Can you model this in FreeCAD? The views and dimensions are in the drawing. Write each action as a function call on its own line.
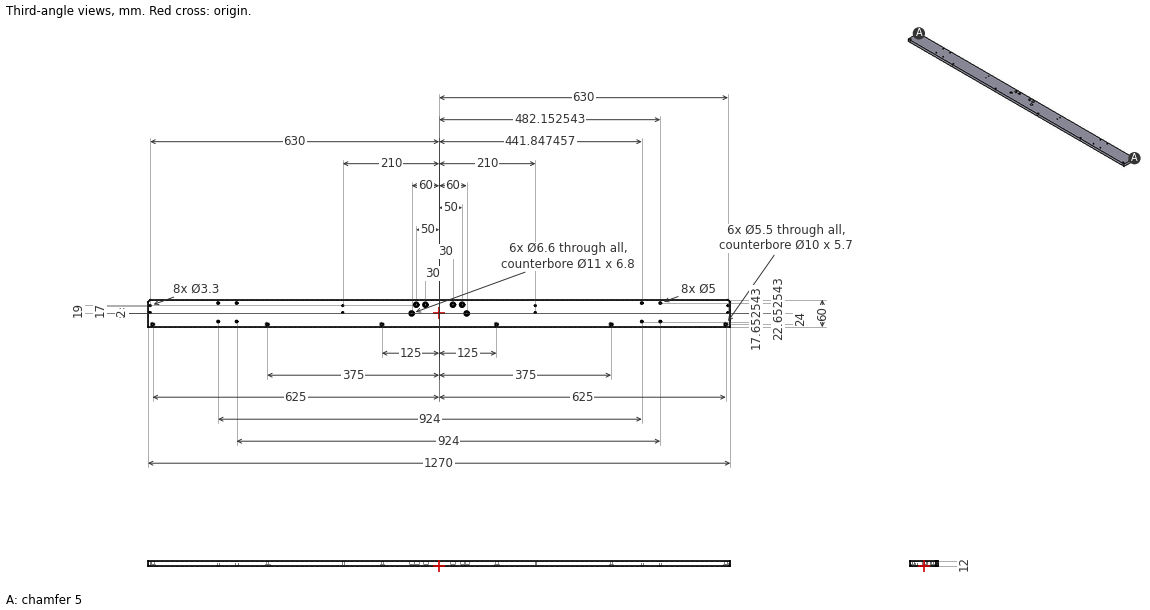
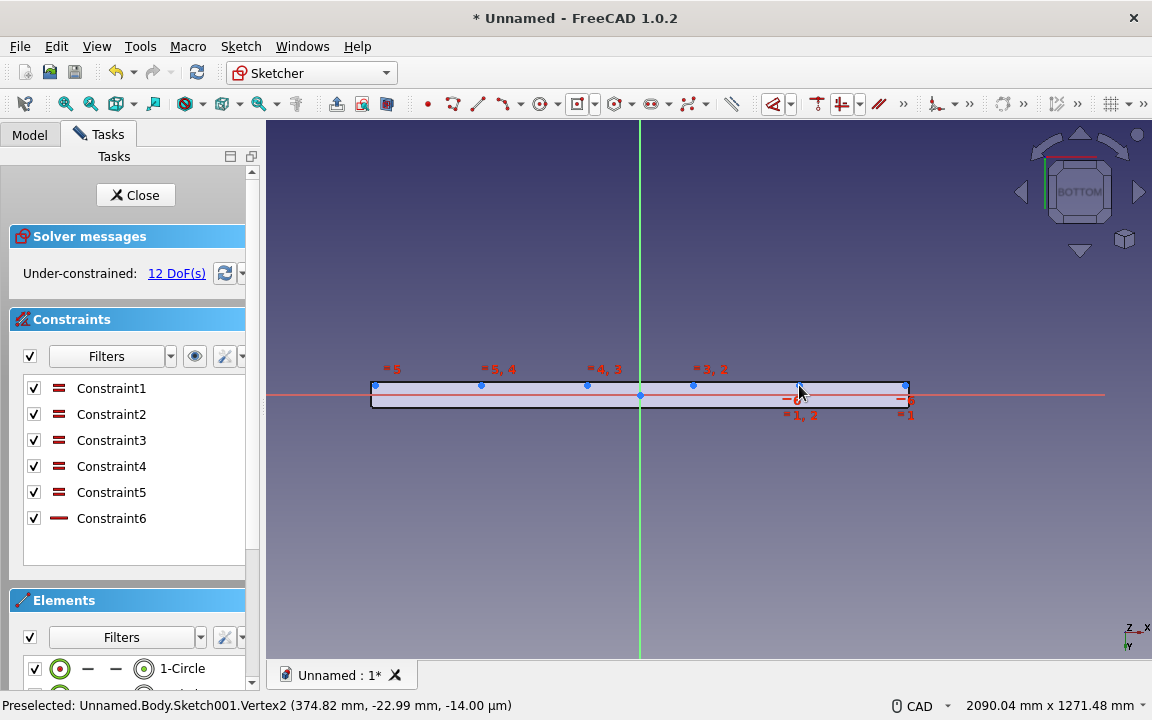
click(799, 386)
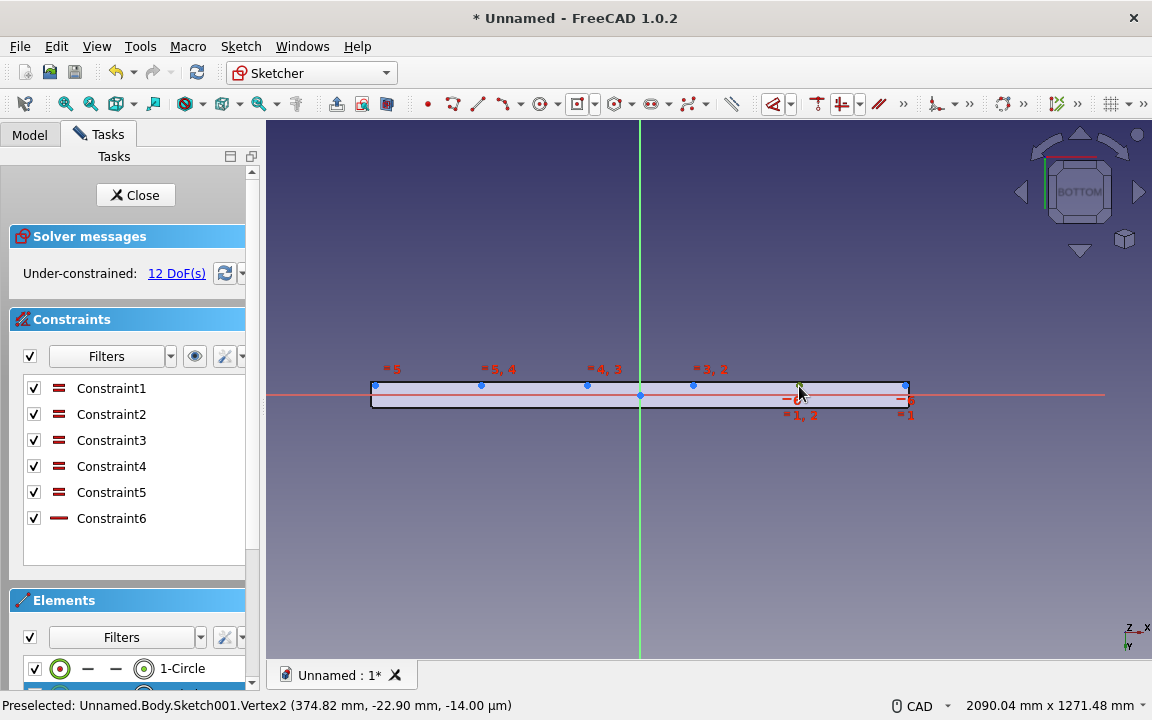
click(693, 385)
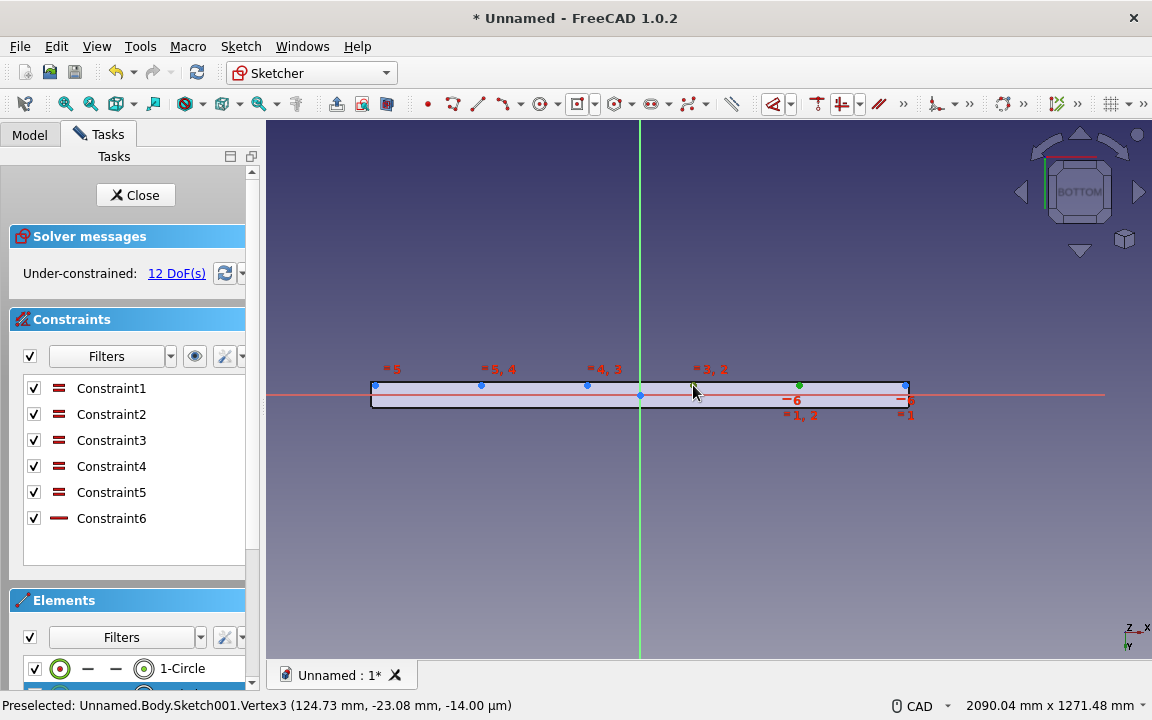
click(860, 104)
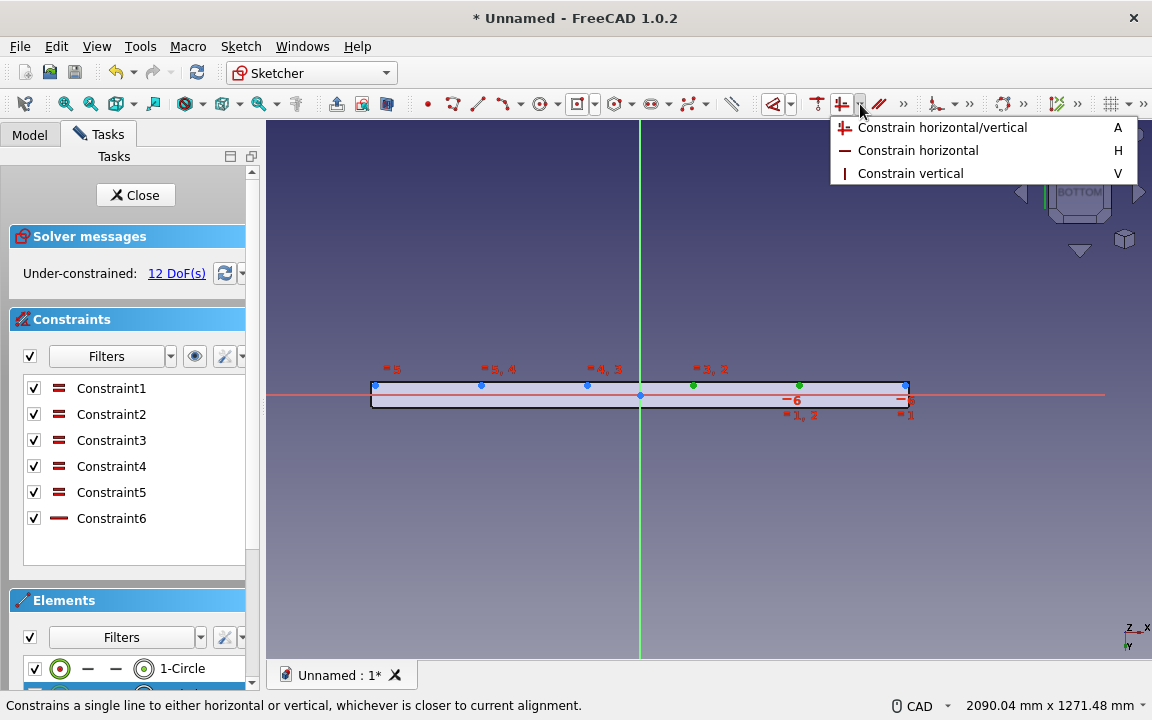
click(984, 150)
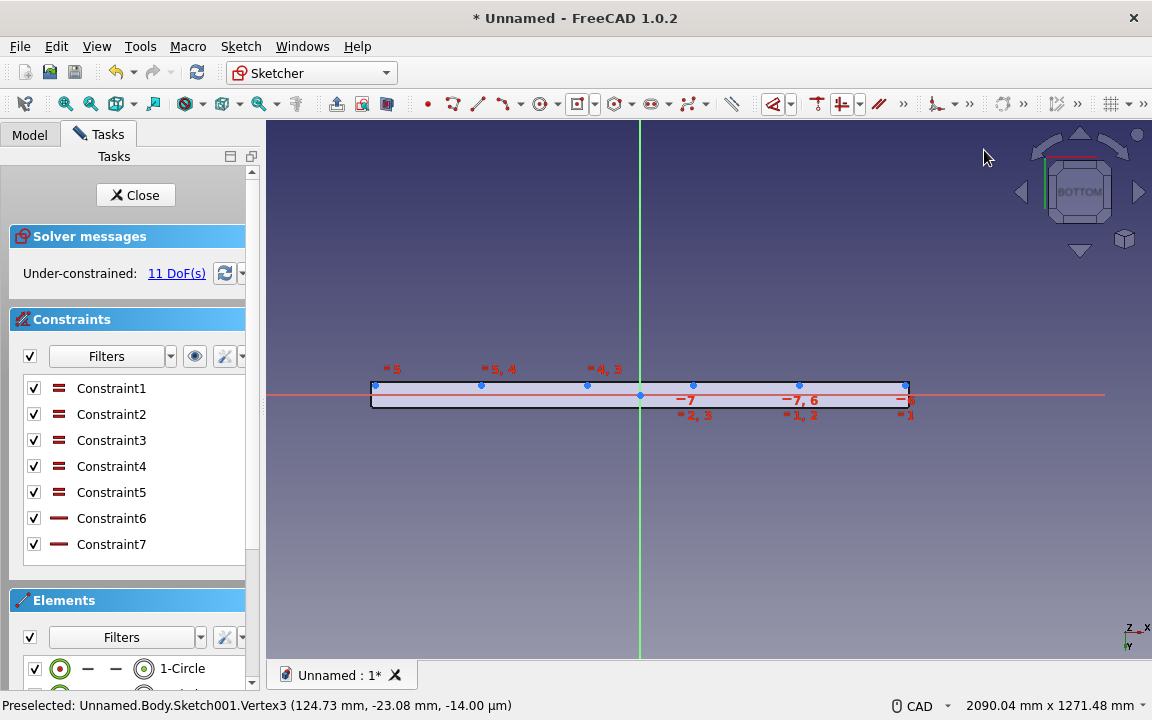
click(693, 386)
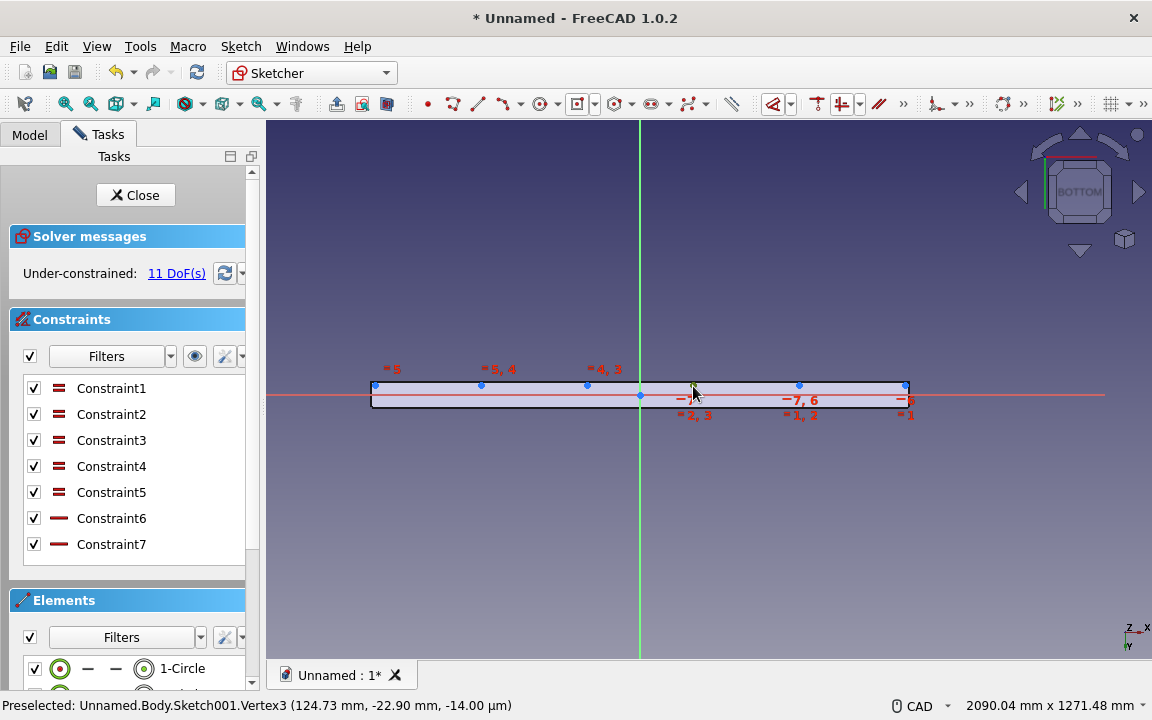
click(587, 385)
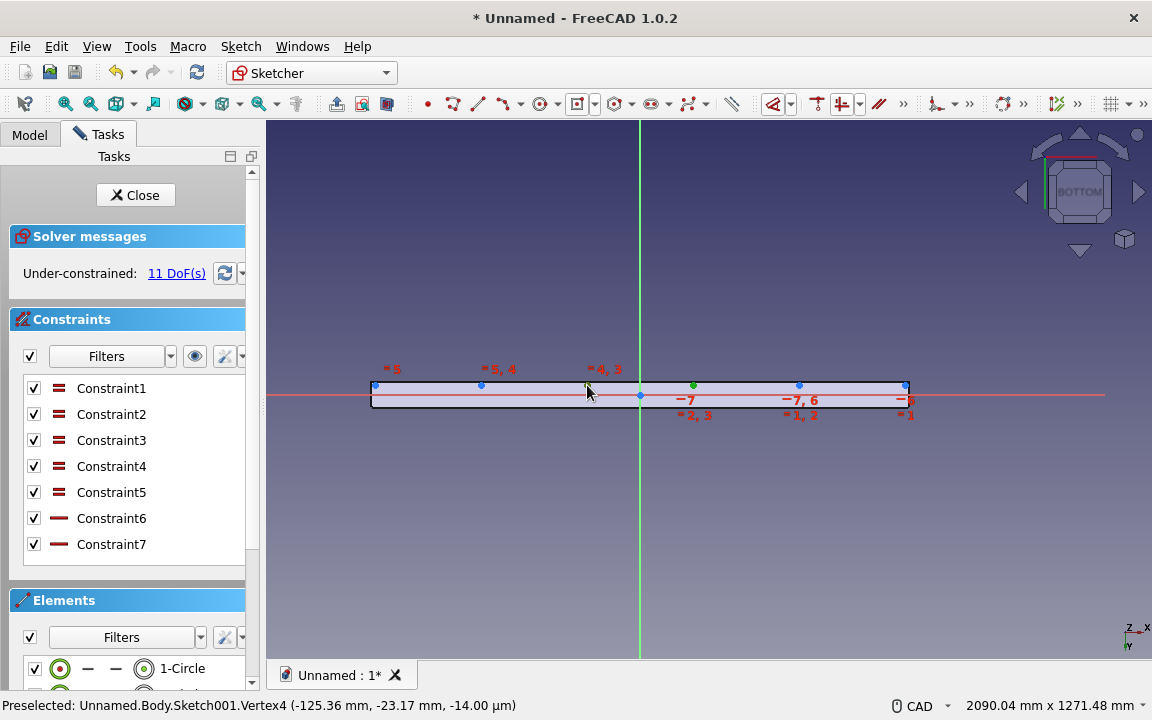
key(h)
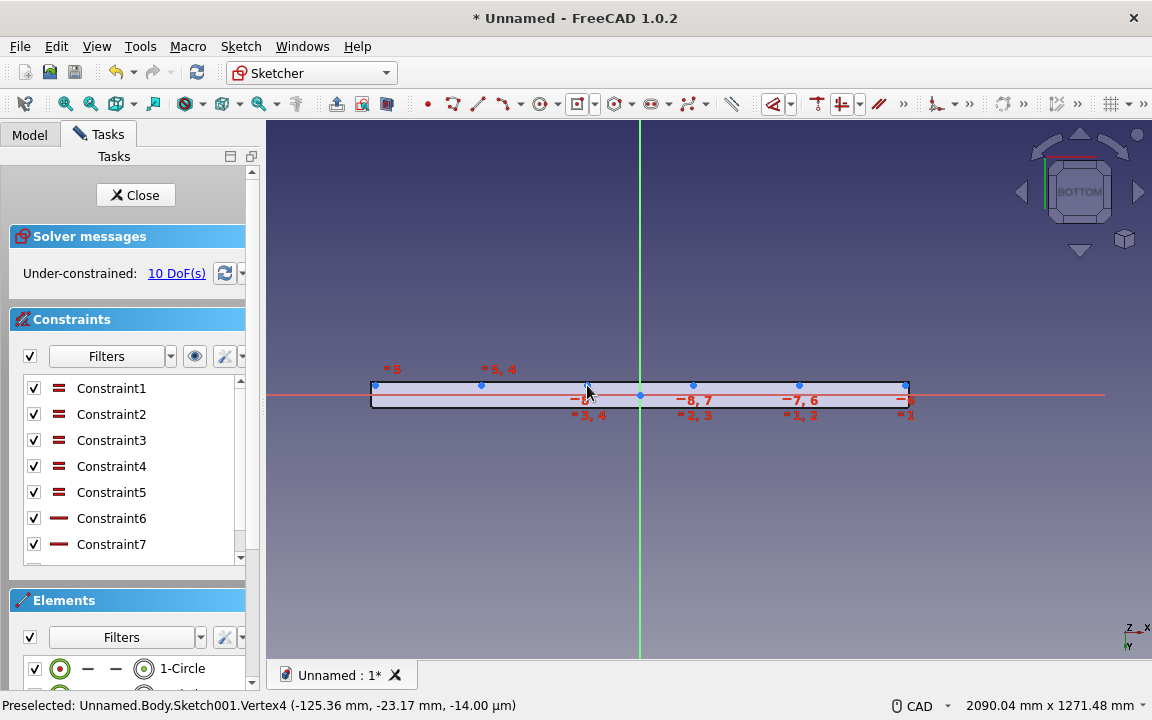
click(587, 386)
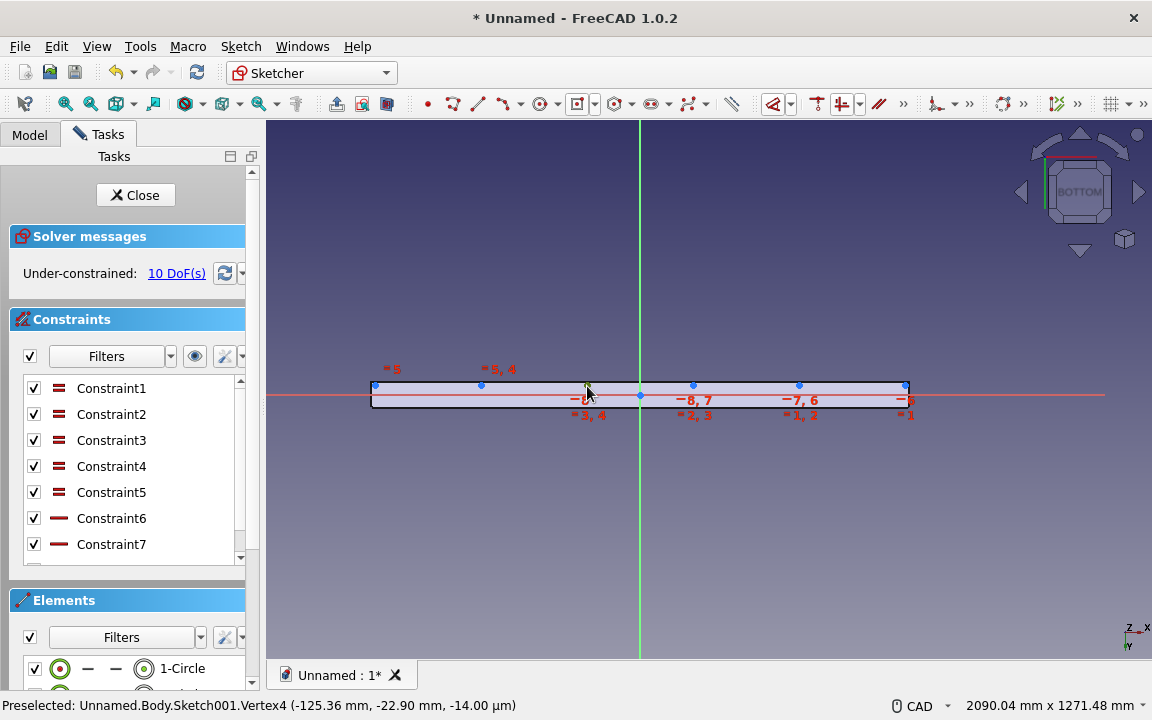
click(481, 385)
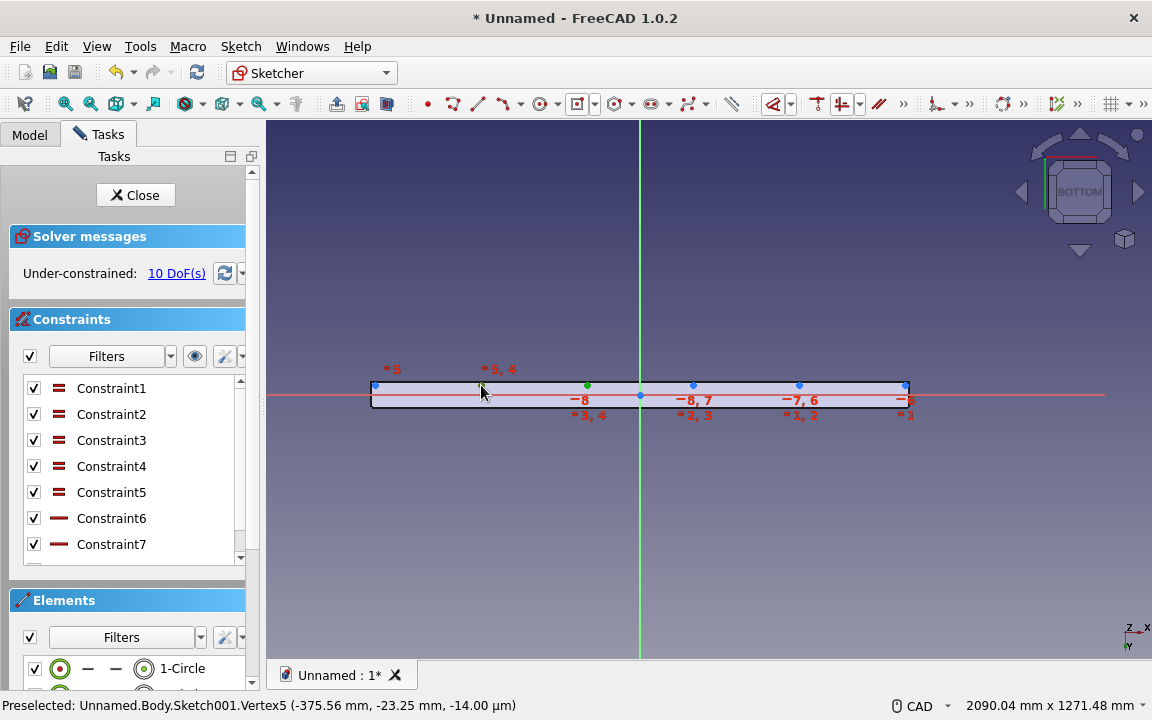
key(h)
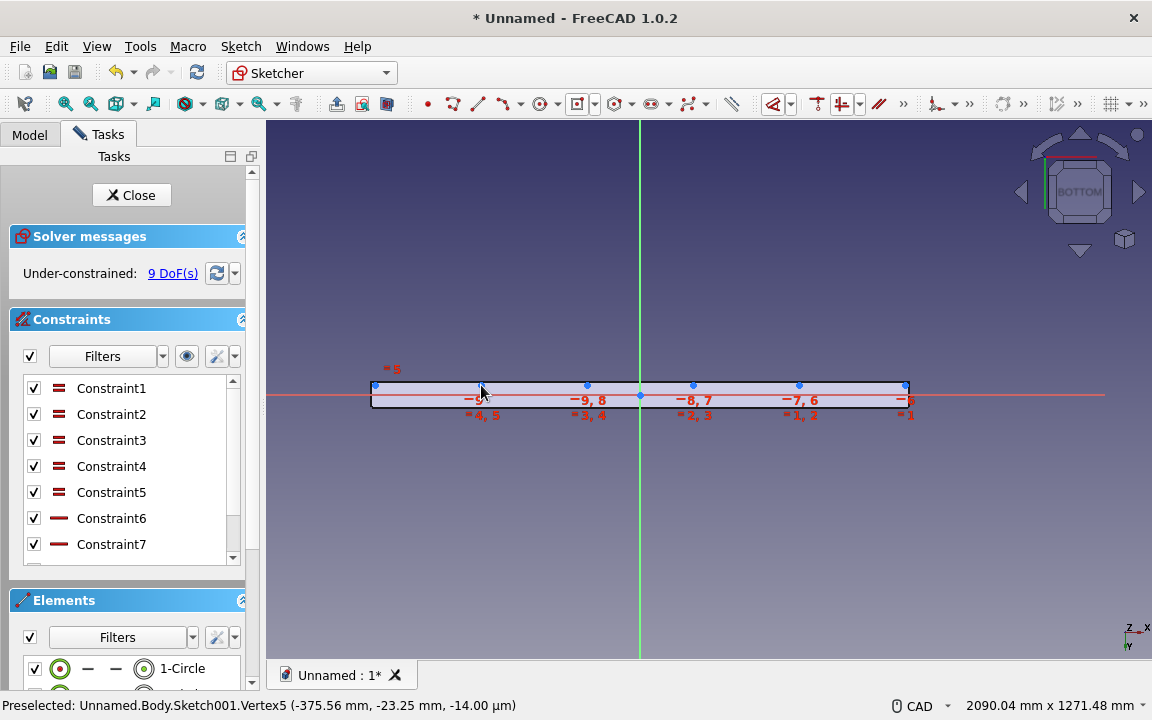
click(481, 386)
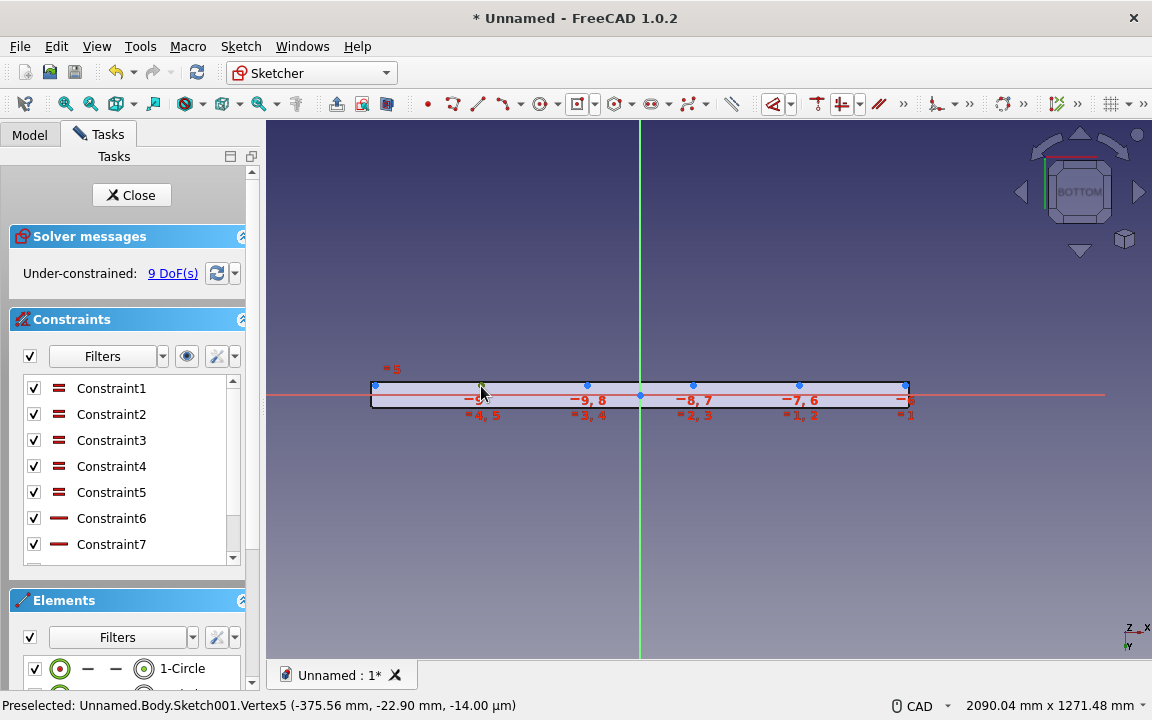
click(376, 386)